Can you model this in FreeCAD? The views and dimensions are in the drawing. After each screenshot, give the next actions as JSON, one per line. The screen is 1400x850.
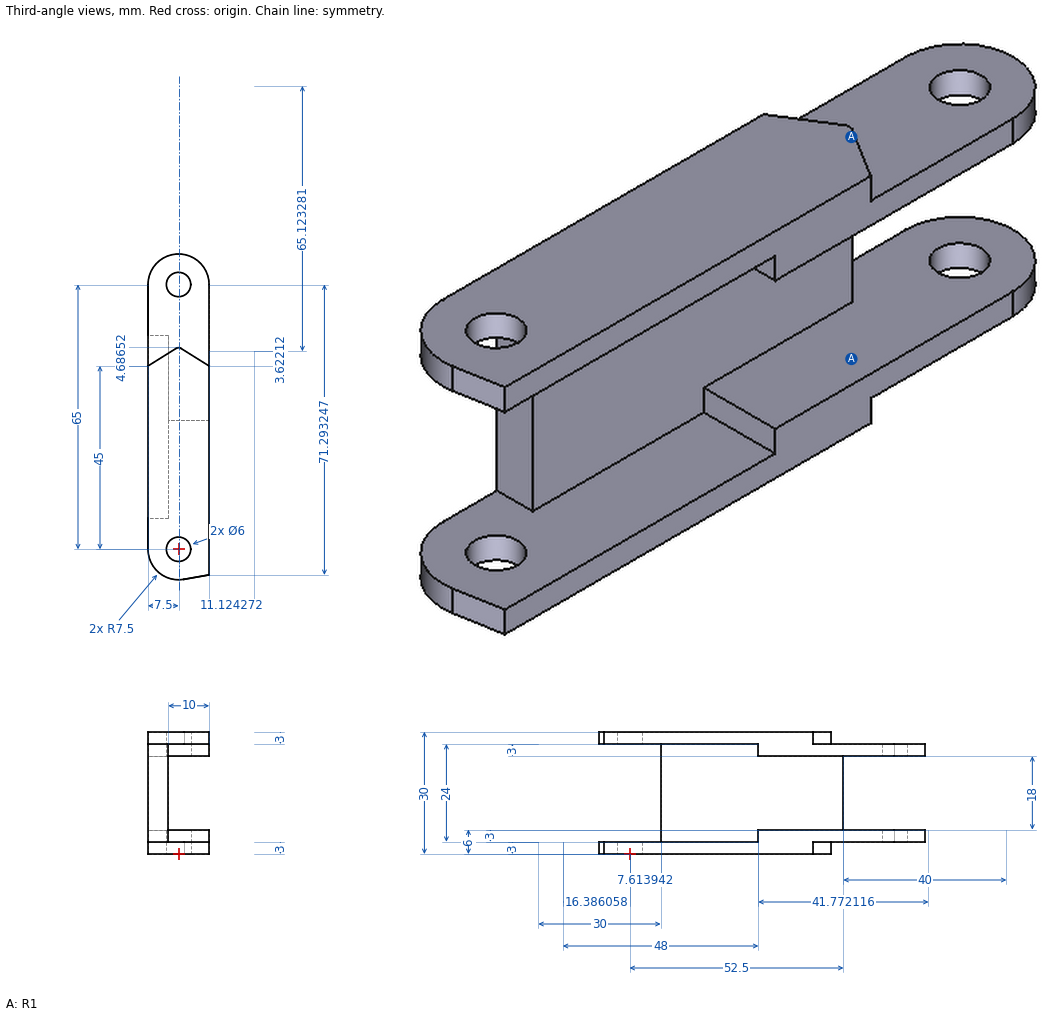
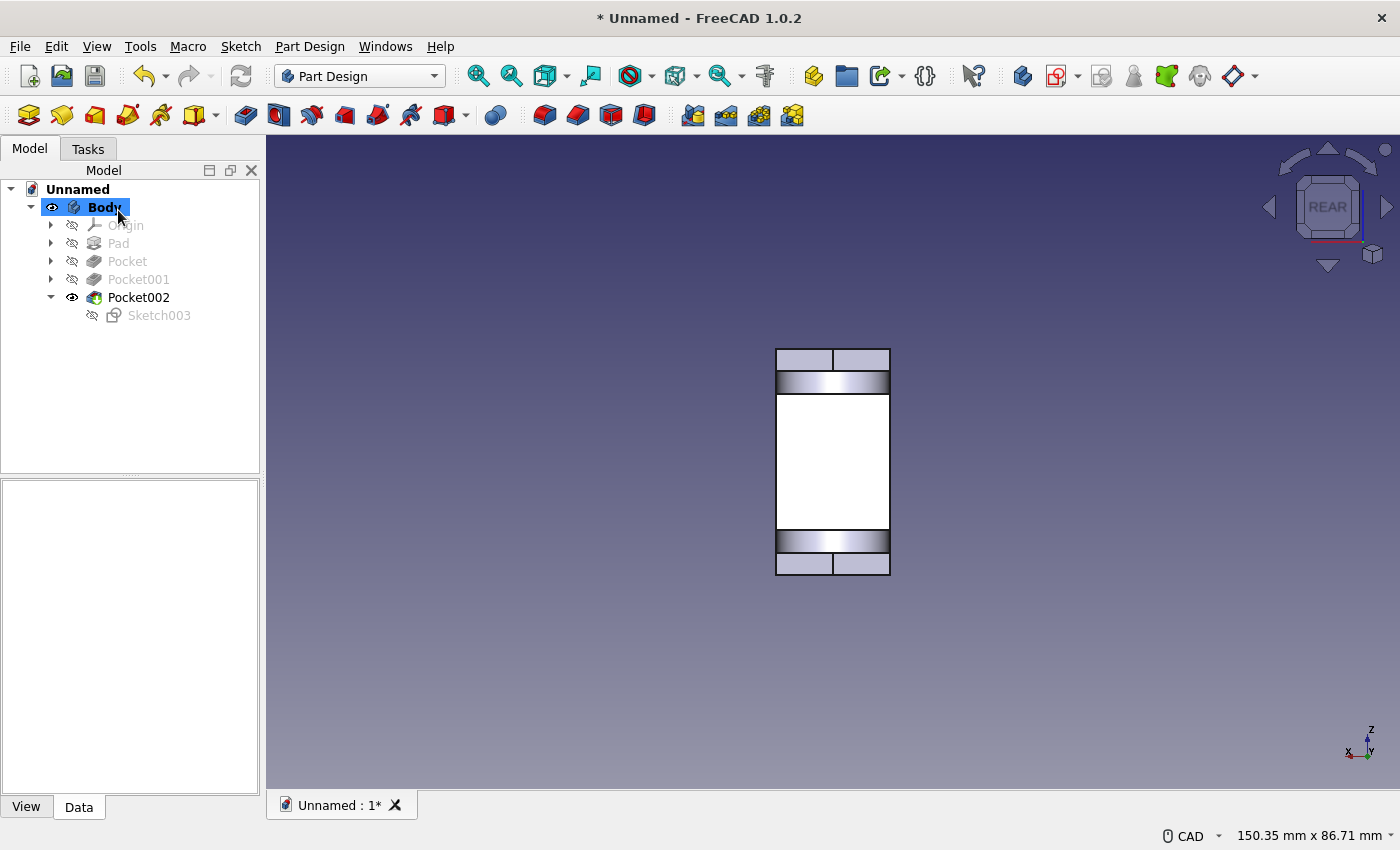
{"action": "left_click", "coordinate": [833, 563]}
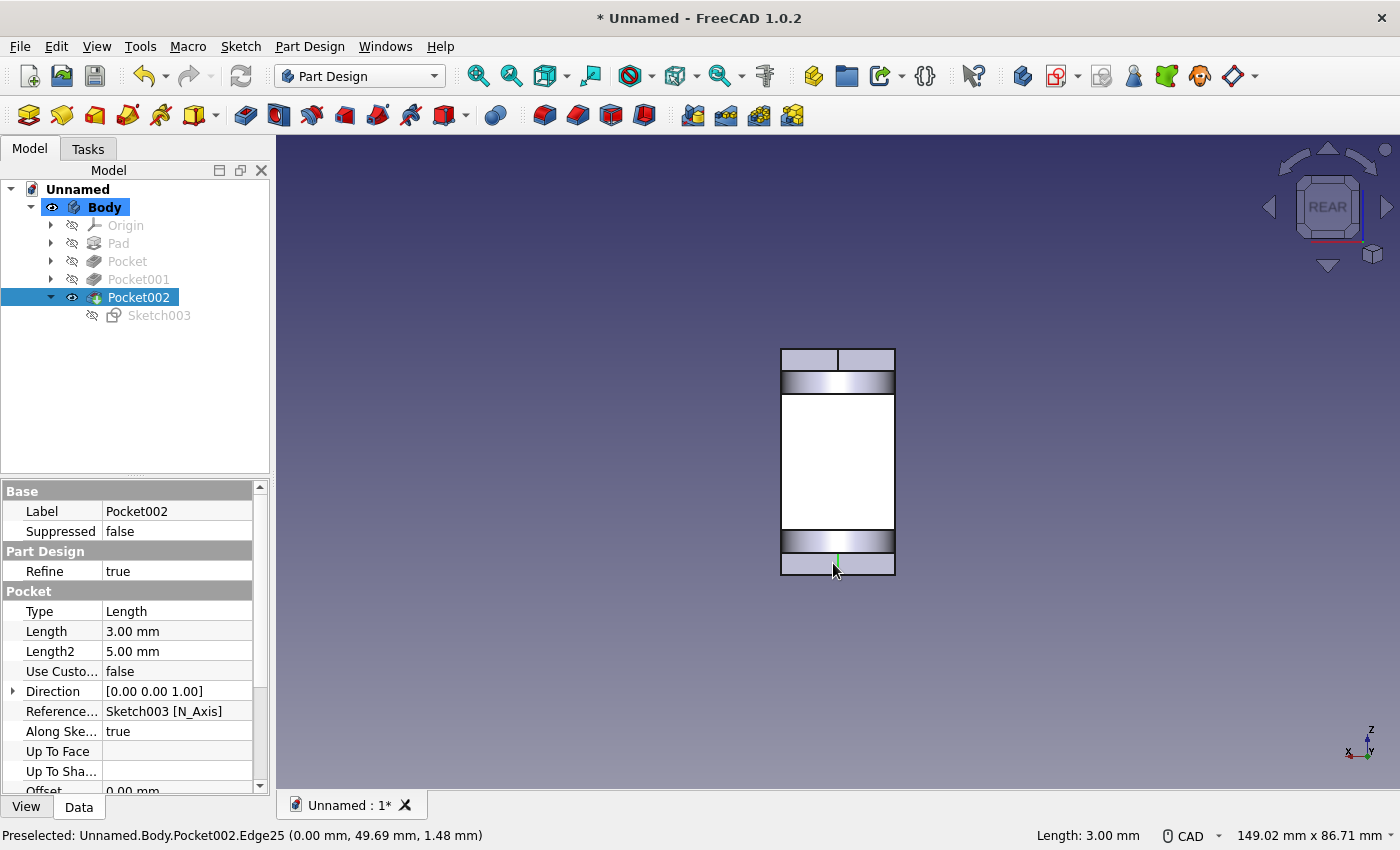
{"action": "left_click", "coordinate": [838, 359], "text": "ctrl"}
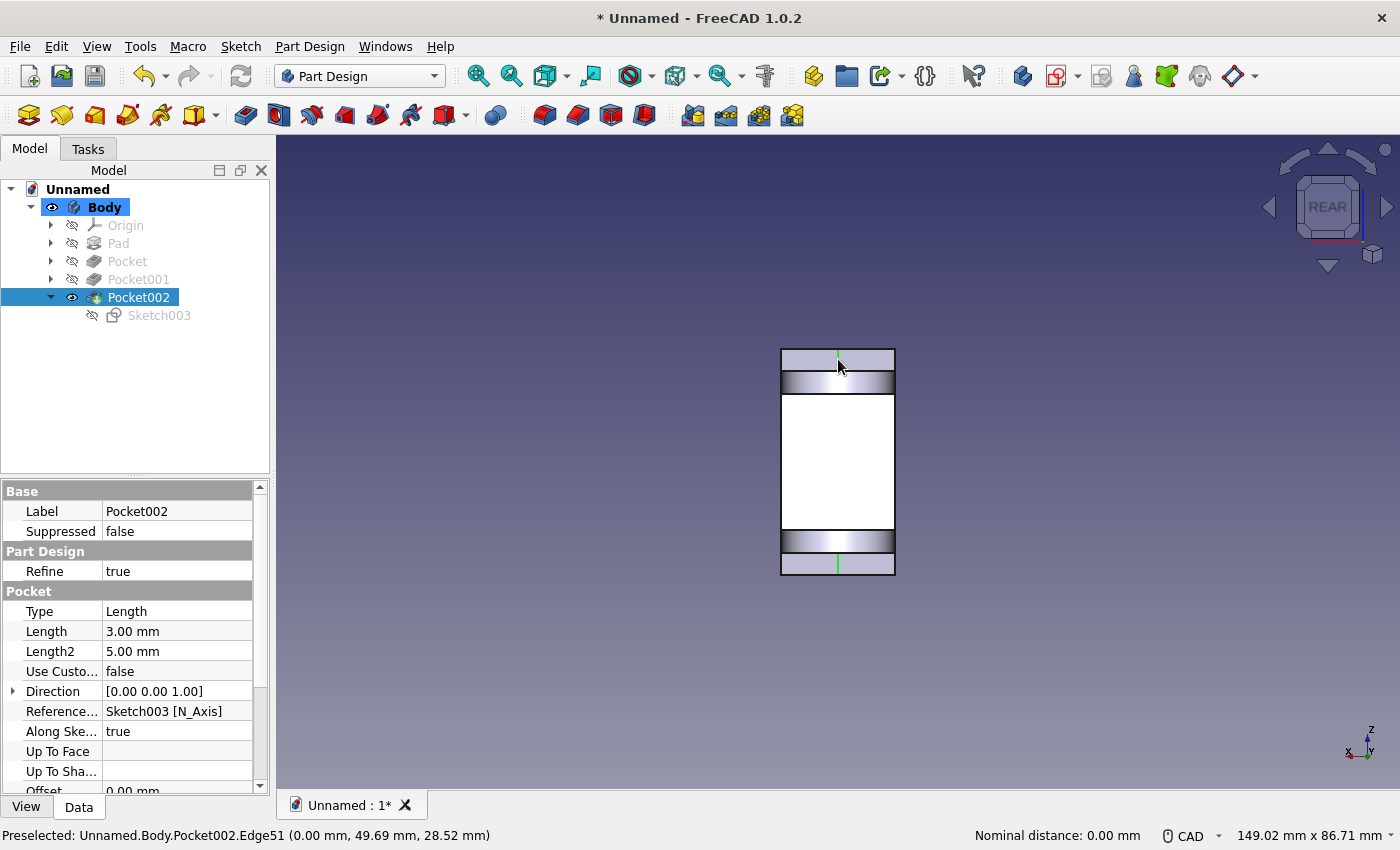
{"action": "left_click", "coordinate": [545, 116]}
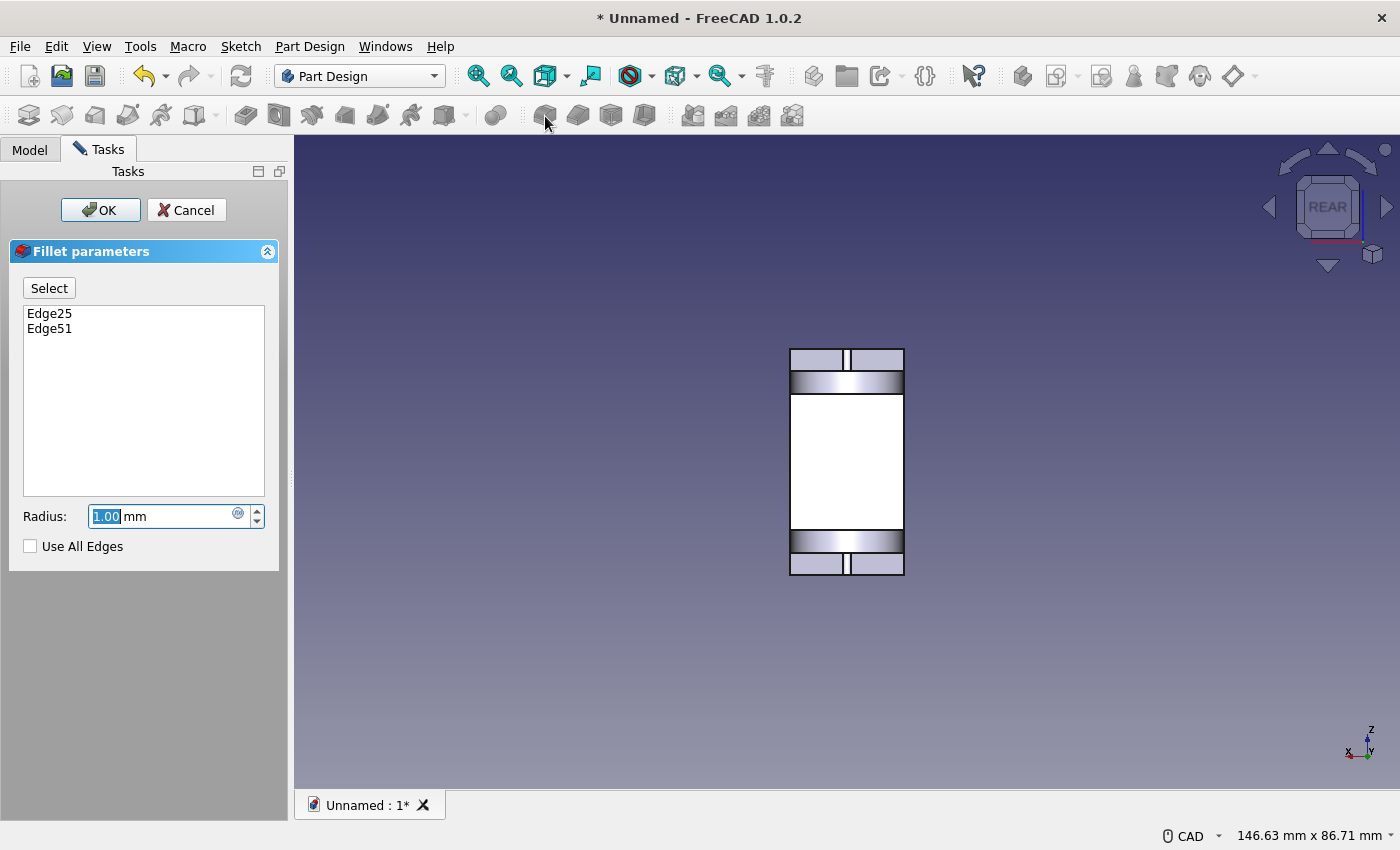
{"action": "type", "text": "1"}
{"action": "key", "text": "Tab"}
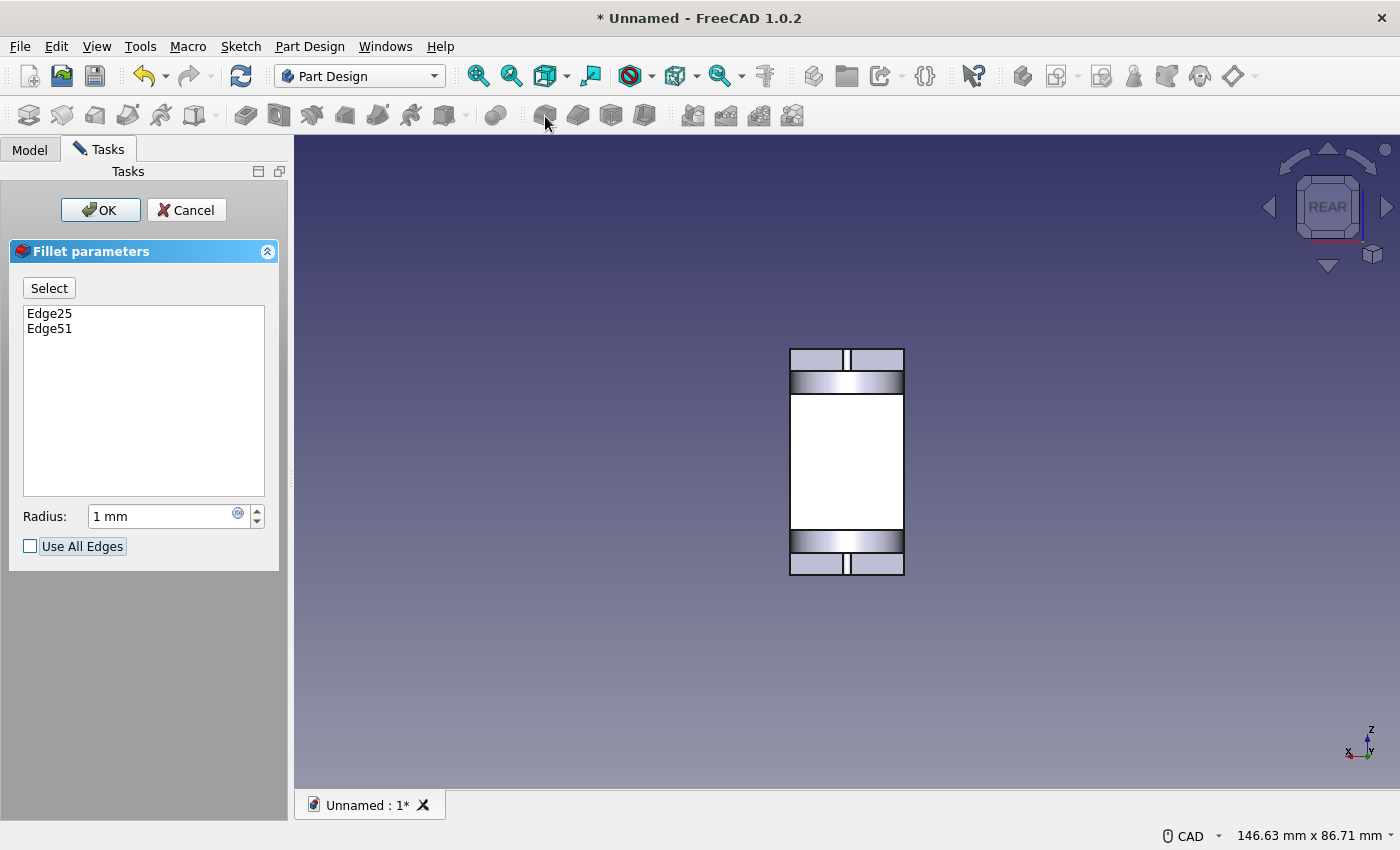
{"action": "left_click", "coordinate": [101, 210]}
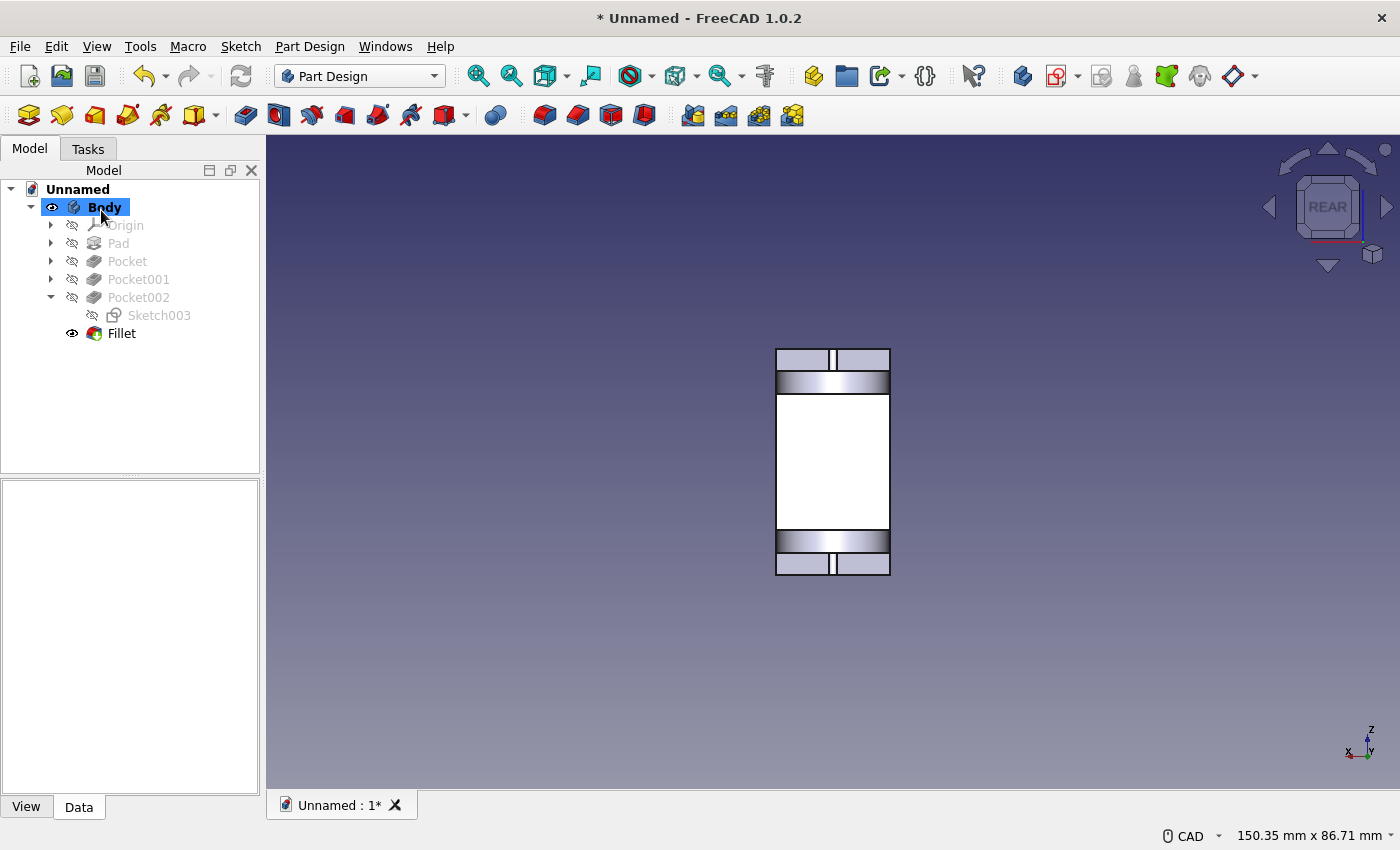
{"action": "key", "text": "v f"}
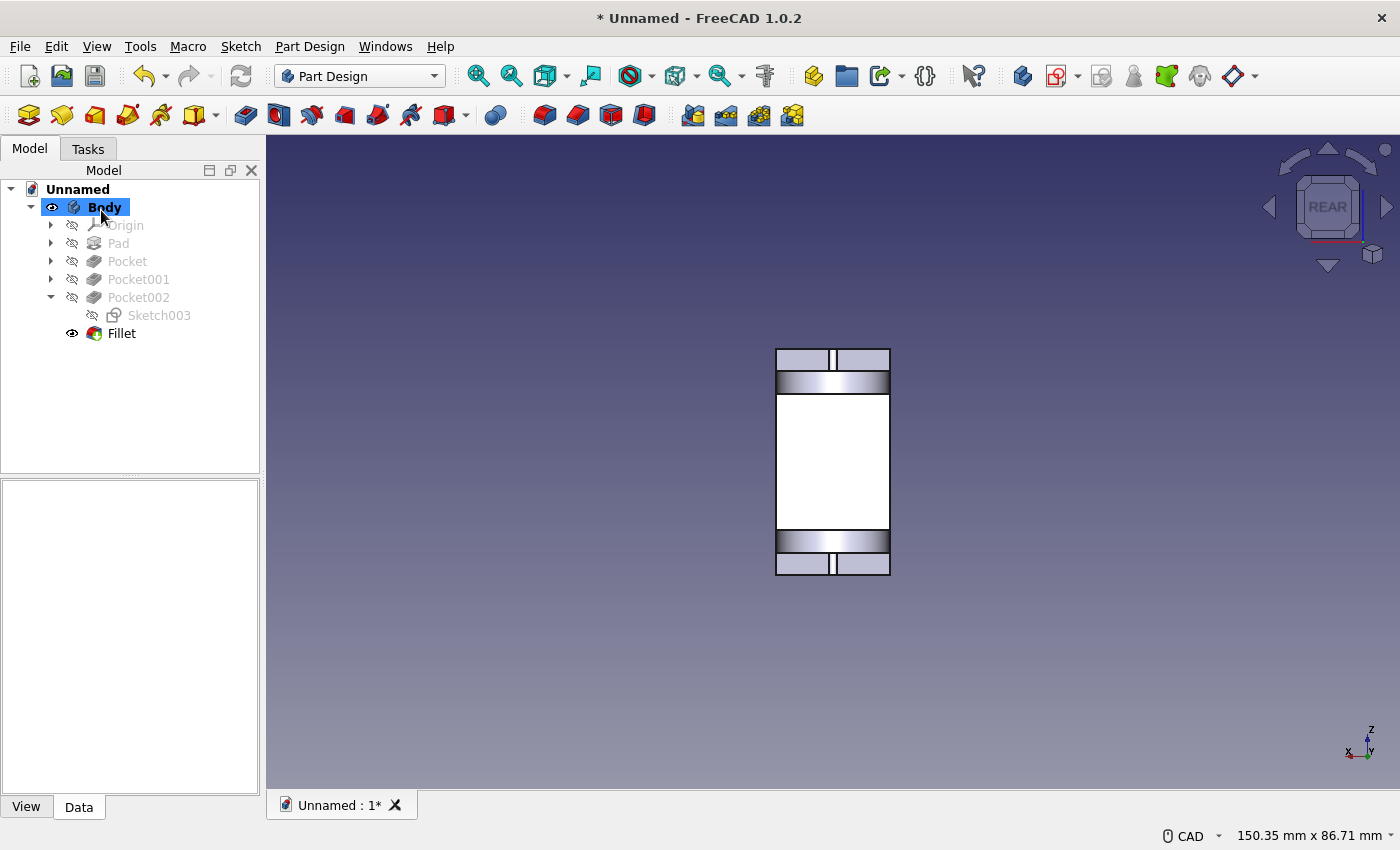
{"action": "key", "text": "0"}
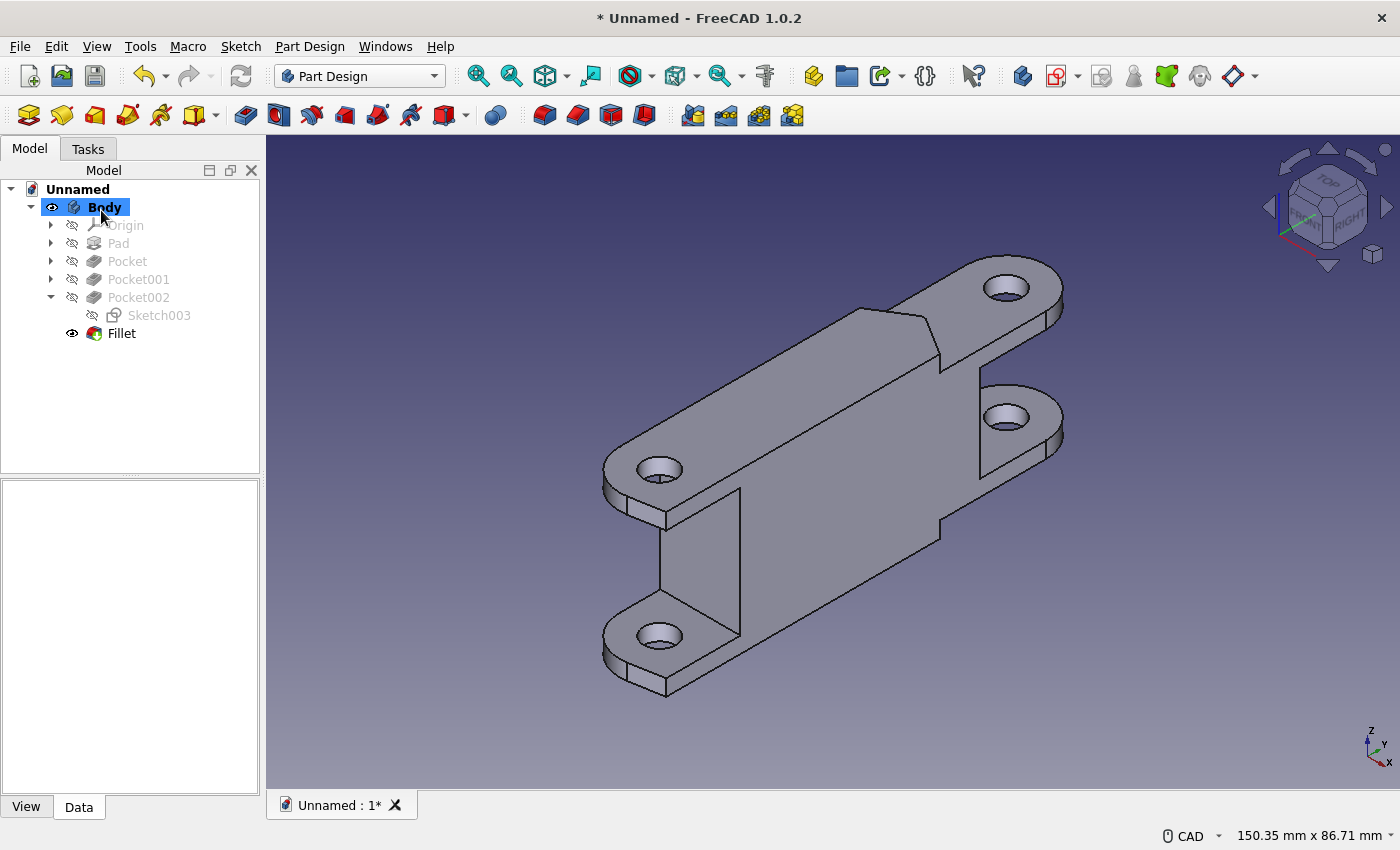
{"action": "left_click", "coordinate": [856, 494]}